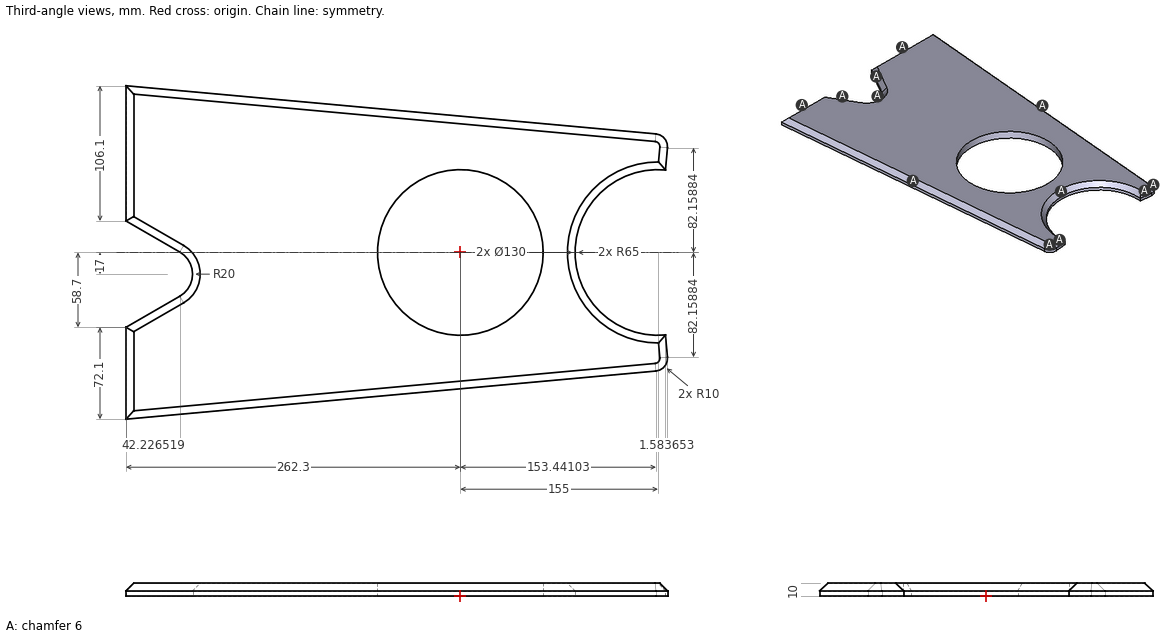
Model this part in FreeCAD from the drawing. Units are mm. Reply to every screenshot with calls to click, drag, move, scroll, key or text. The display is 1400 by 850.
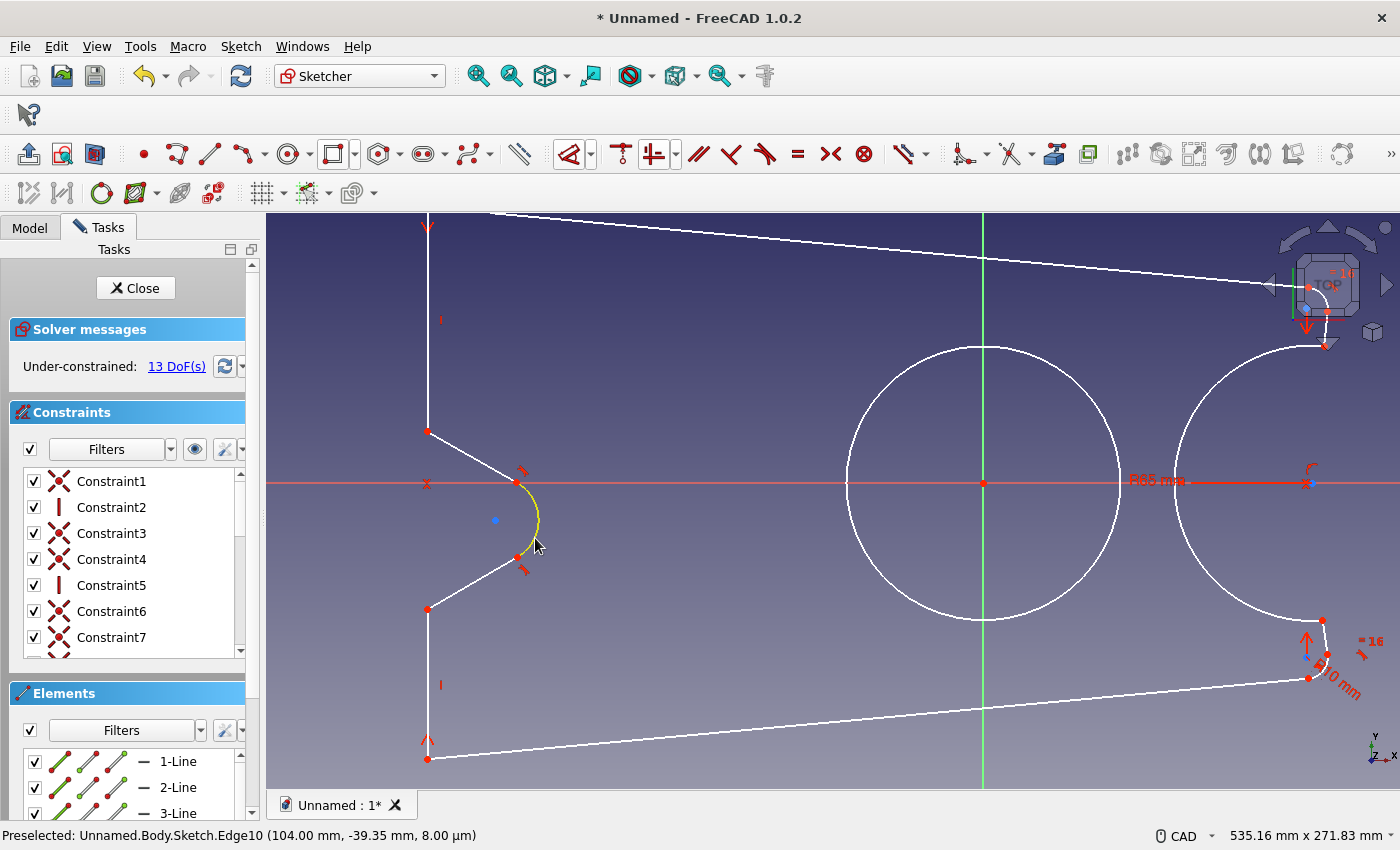
click(535, 537)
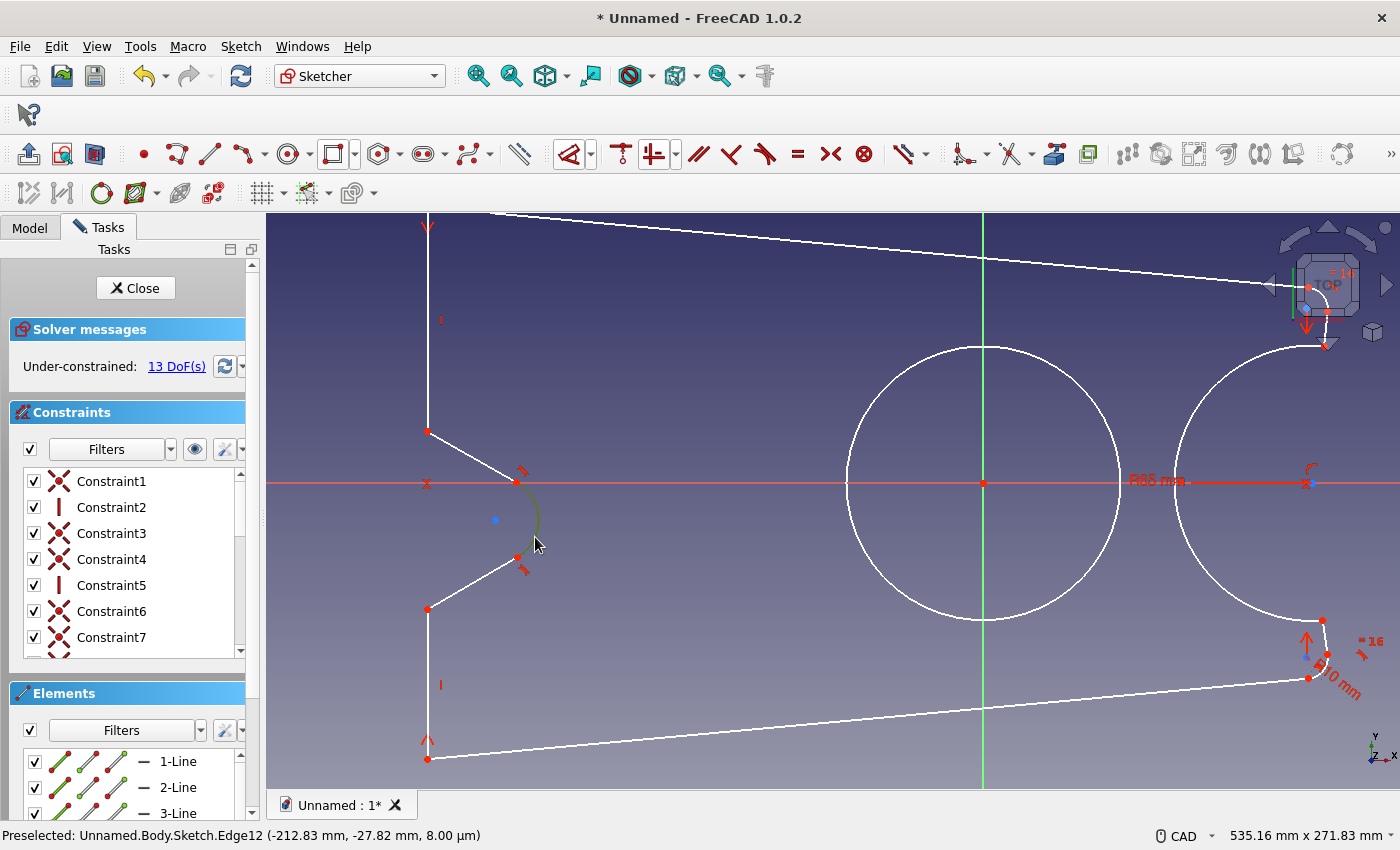
click(590, 154)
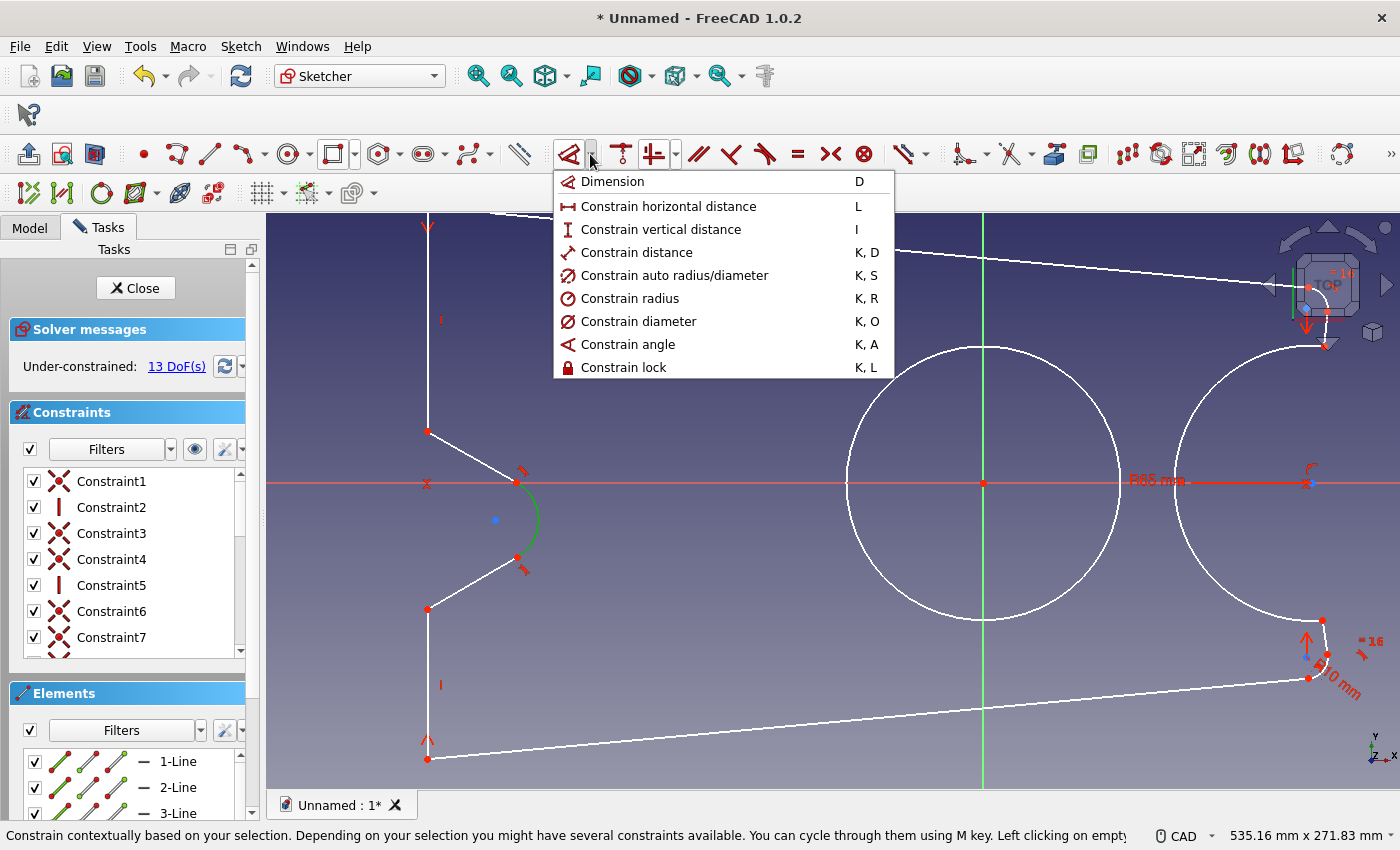
click(724, 298)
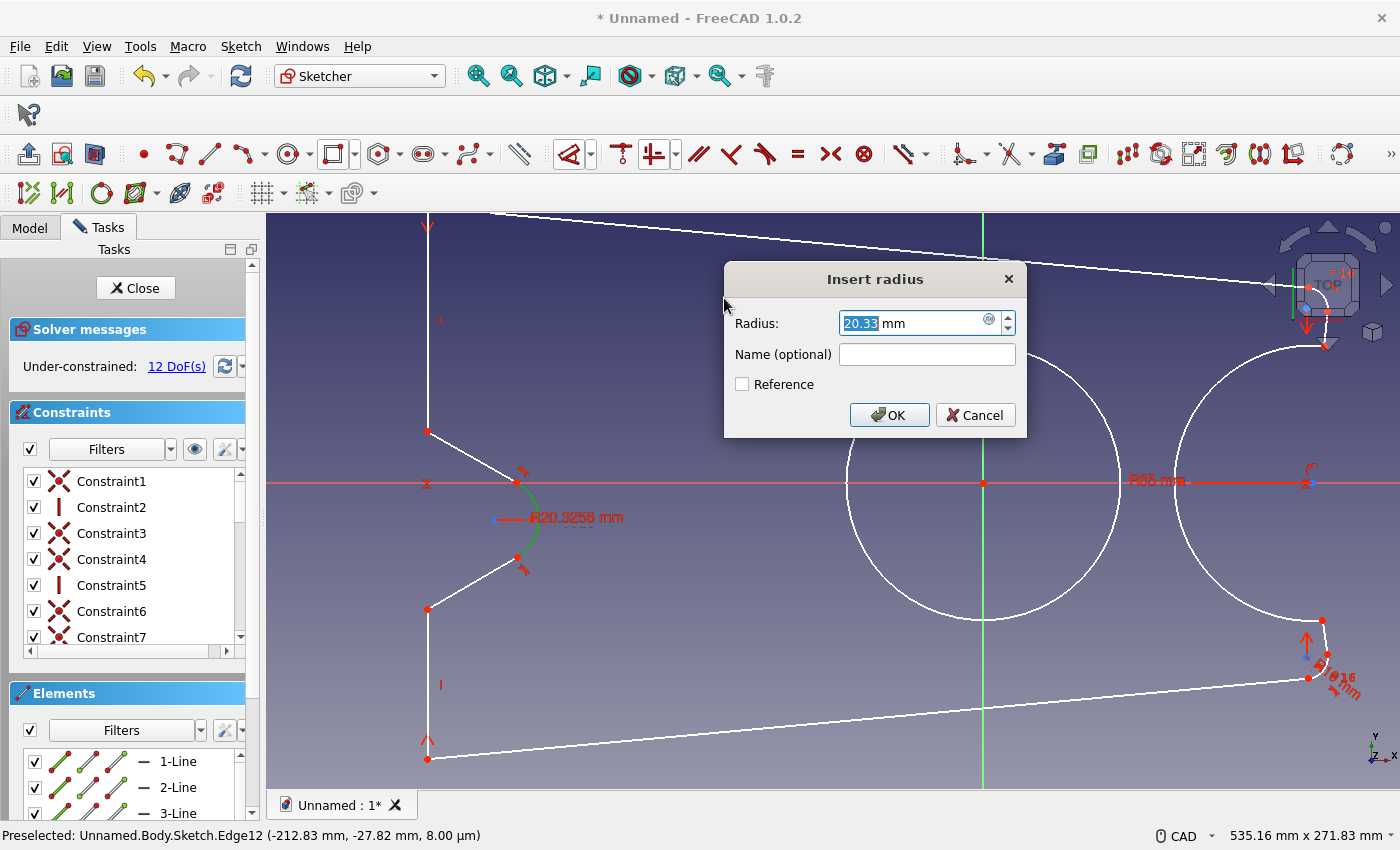
text(20)
key(Return)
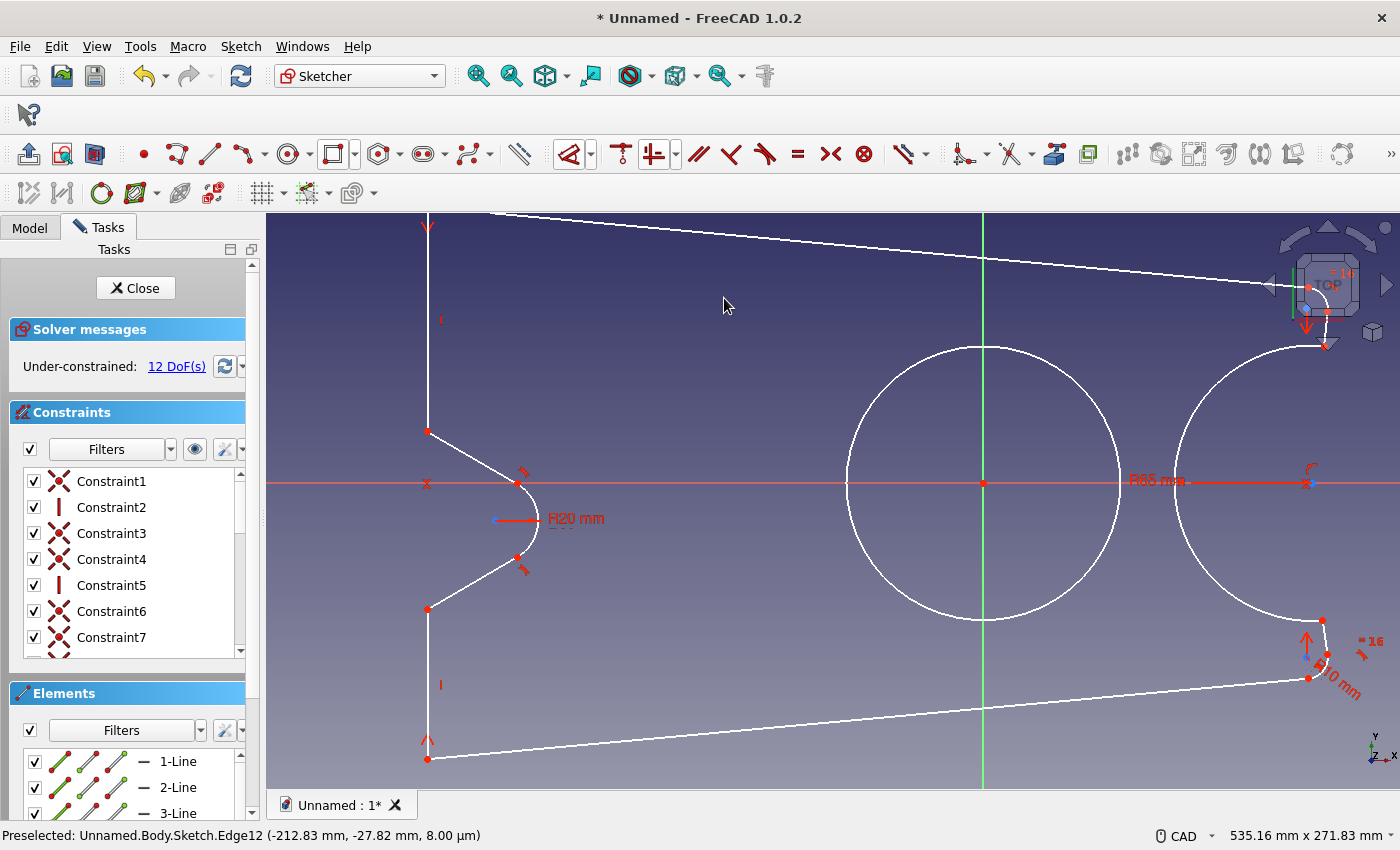
click(1080, 386)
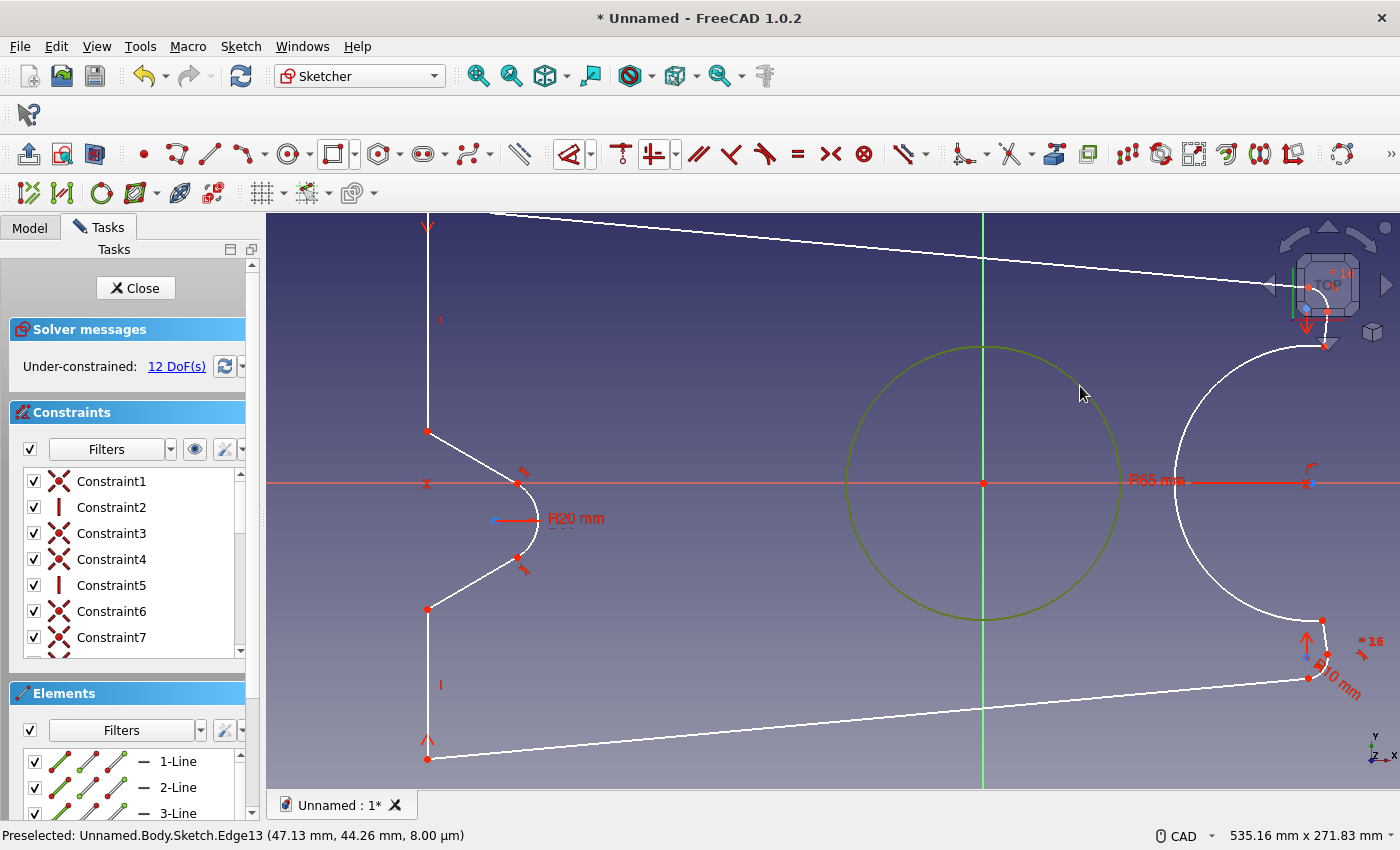
key(k)
key(o)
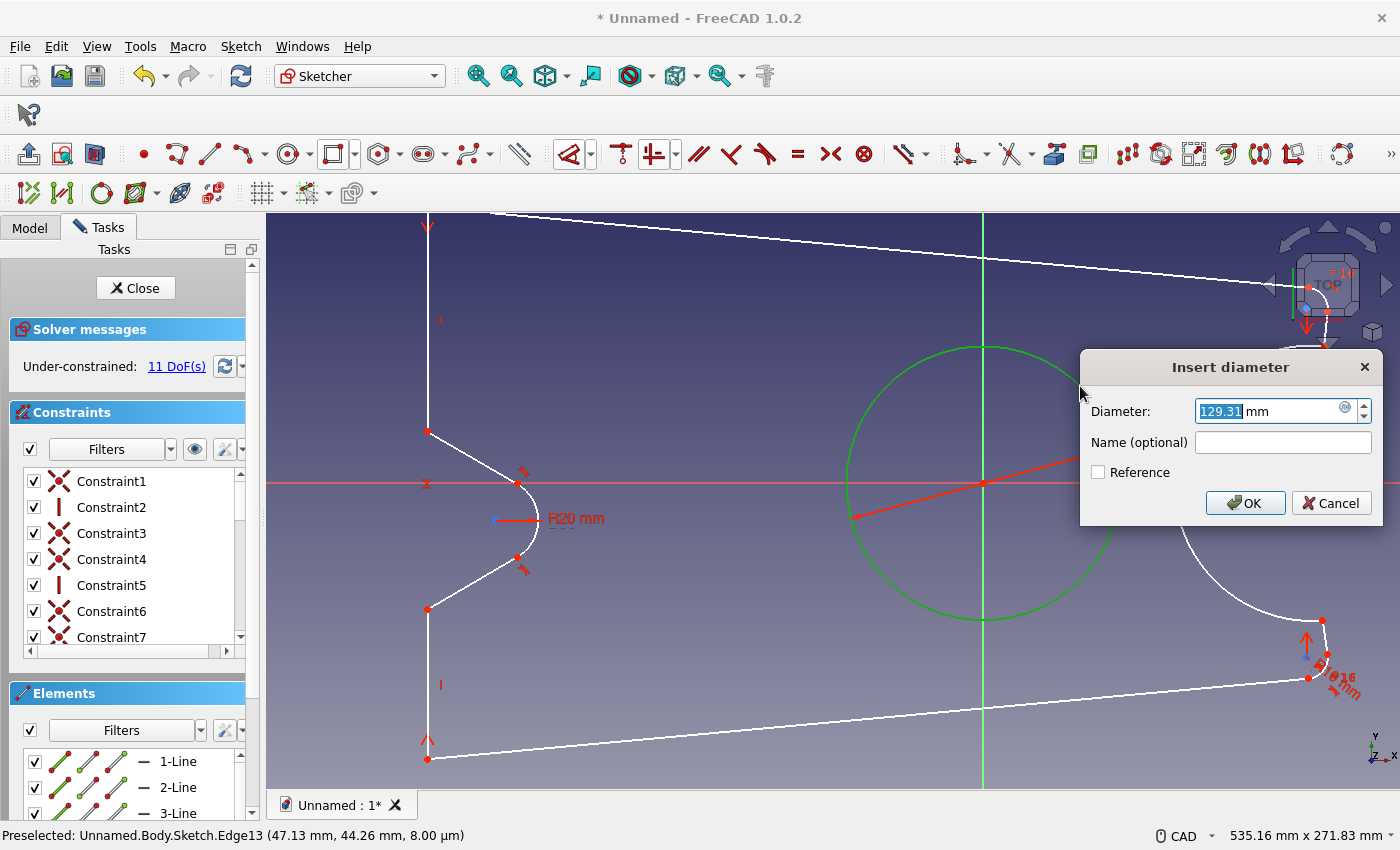
text(130)
key(Return)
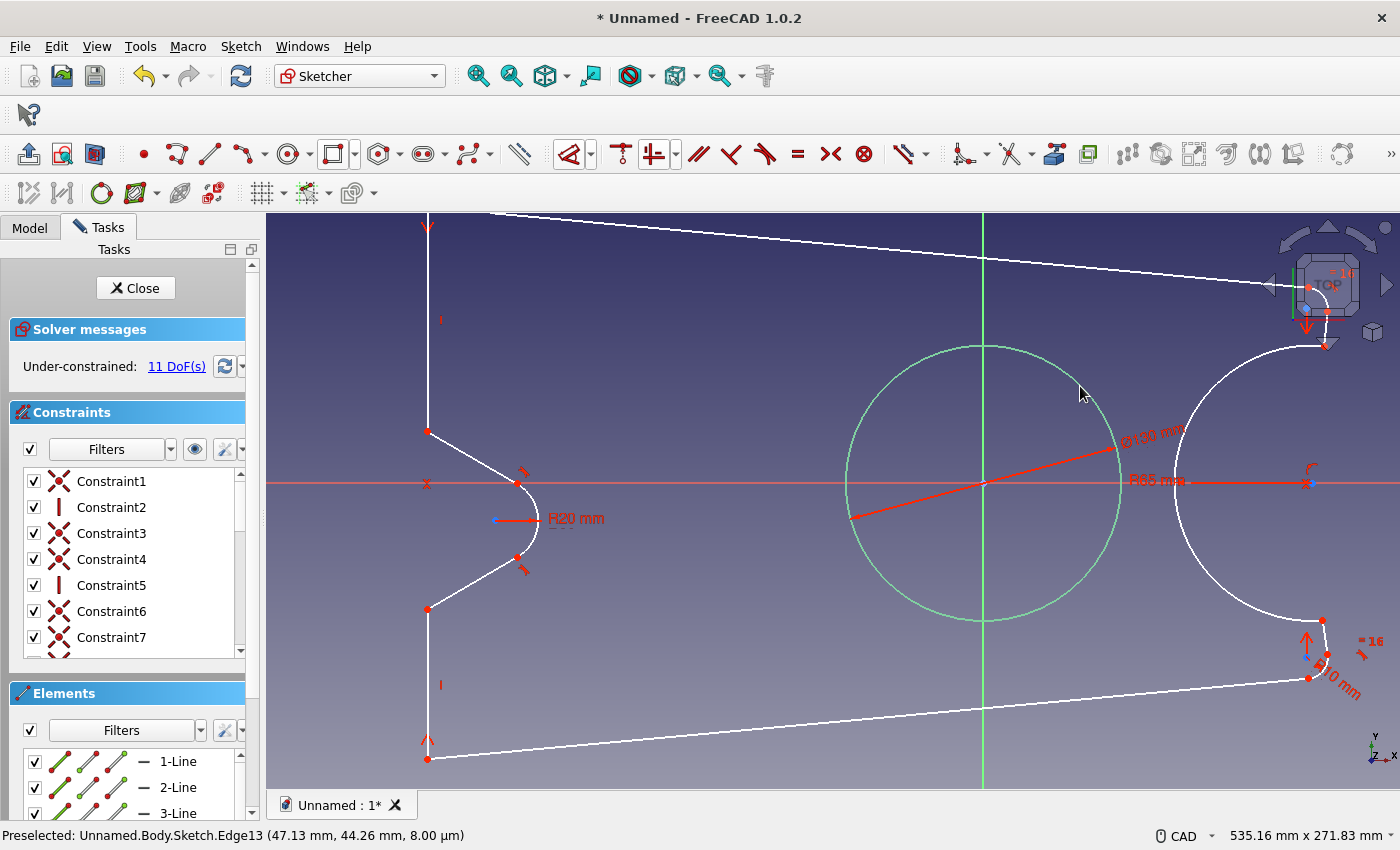
click(496, 521)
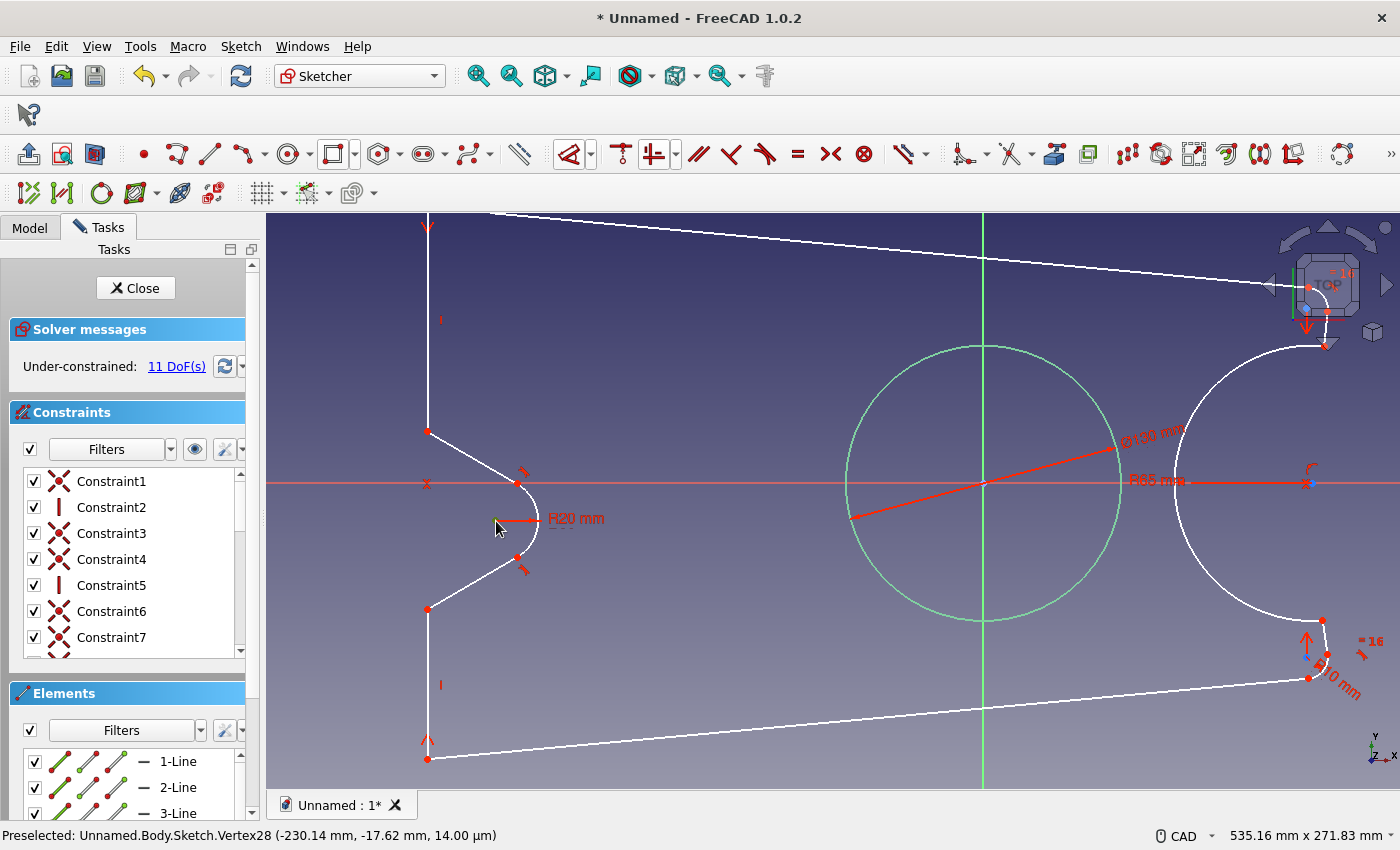
key(i)